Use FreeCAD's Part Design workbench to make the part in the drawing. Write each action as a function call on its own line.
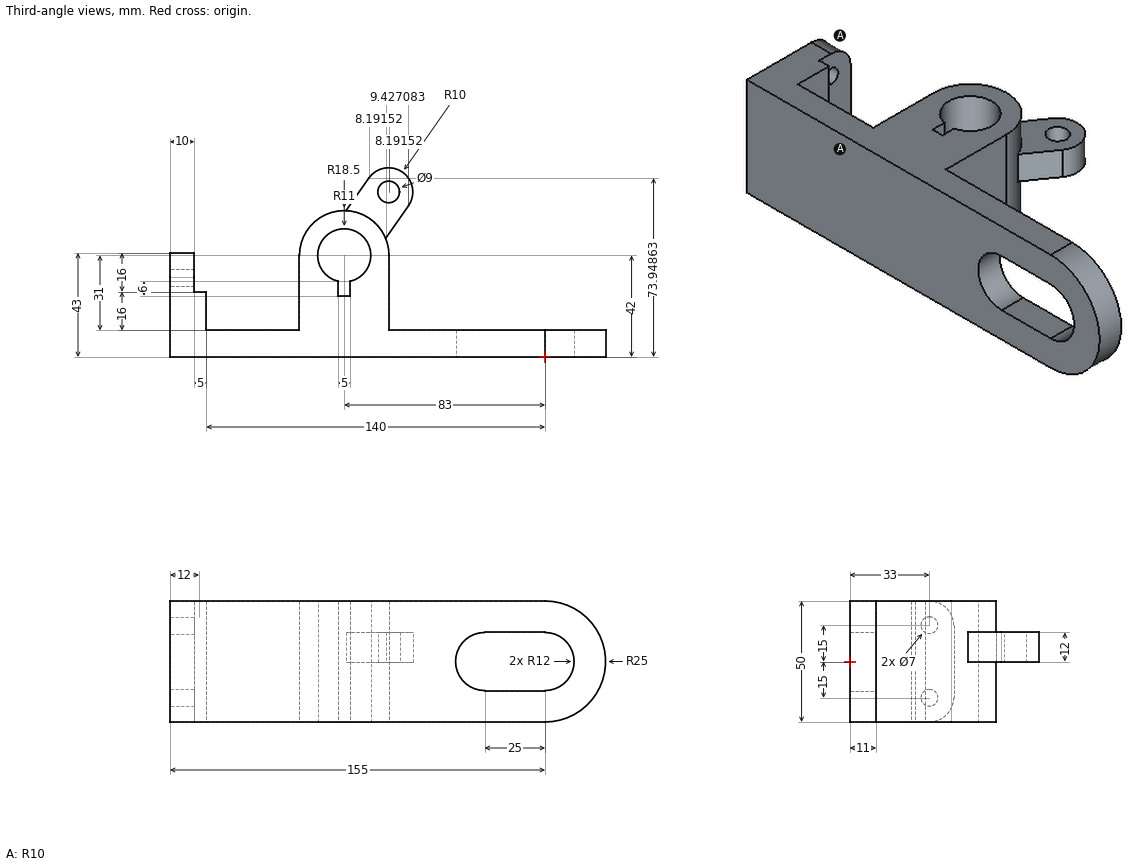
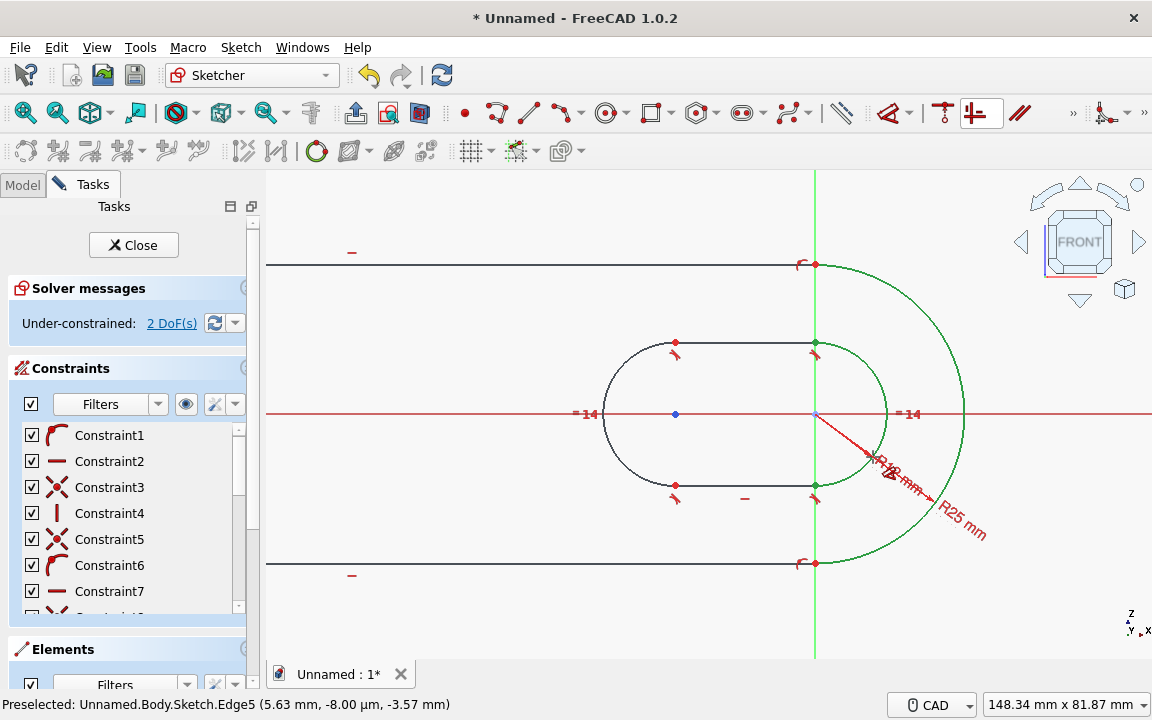
click(773, 486)
click(745, 520)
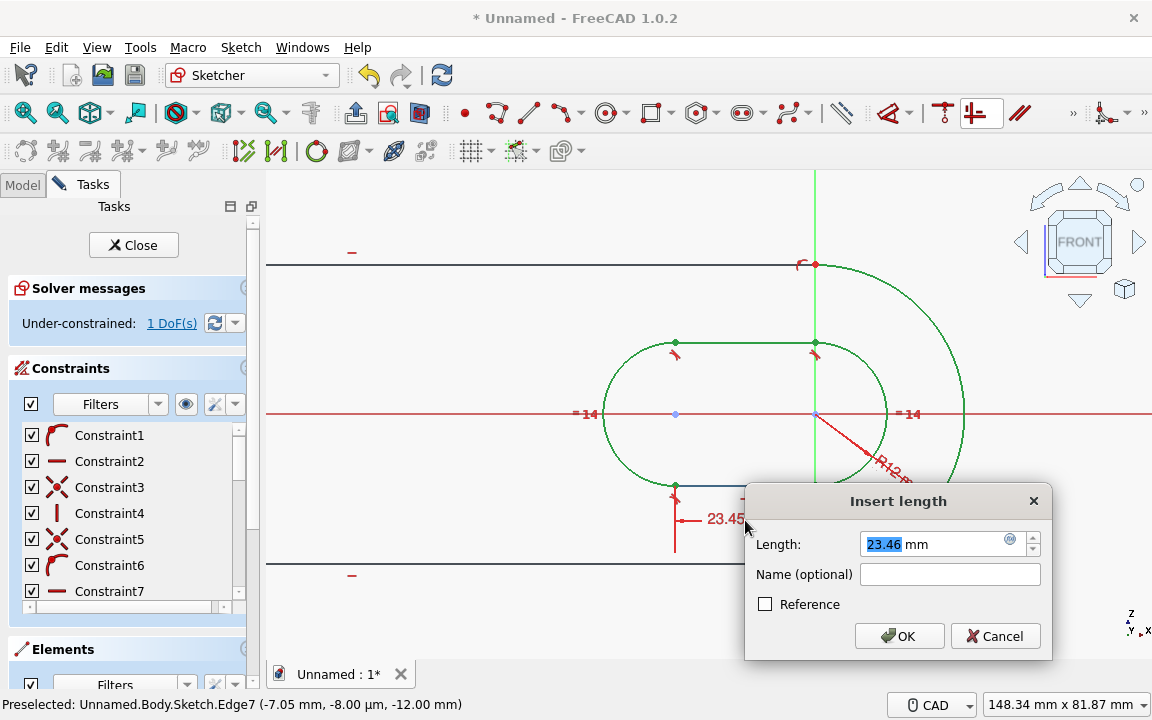
text(25)
key(Return)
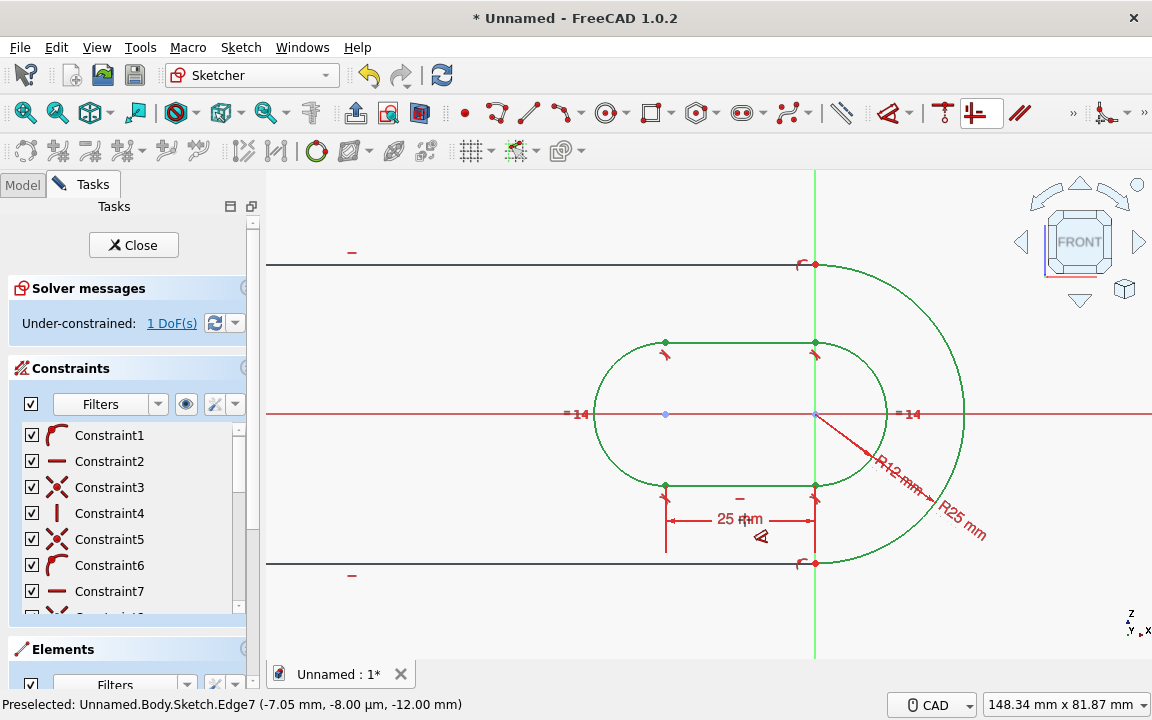
click(537, 564)
click(555, 598)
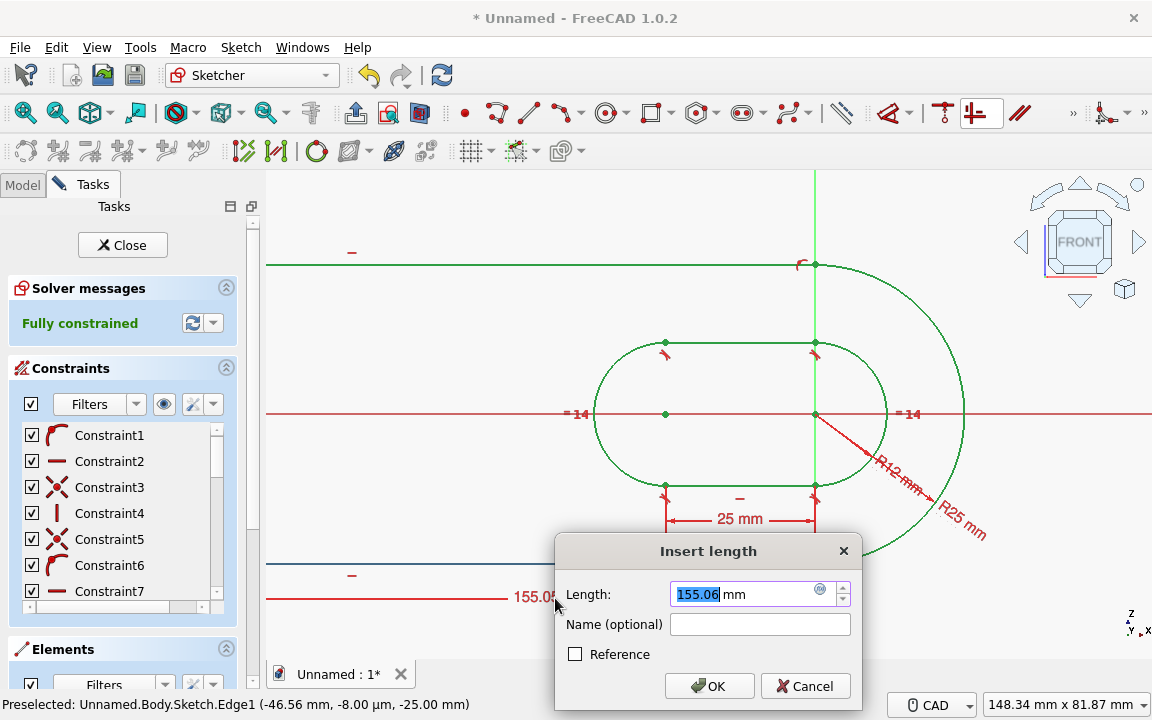
text(155)
key(Return)
key(Escape)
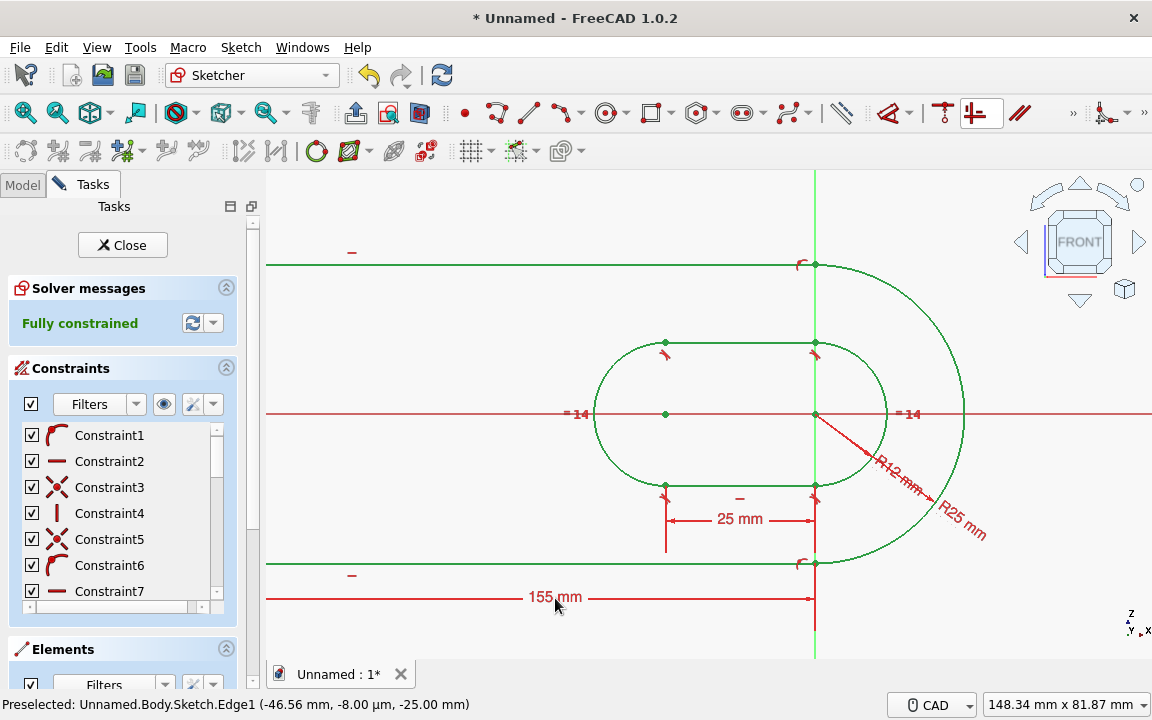
click(123, 245)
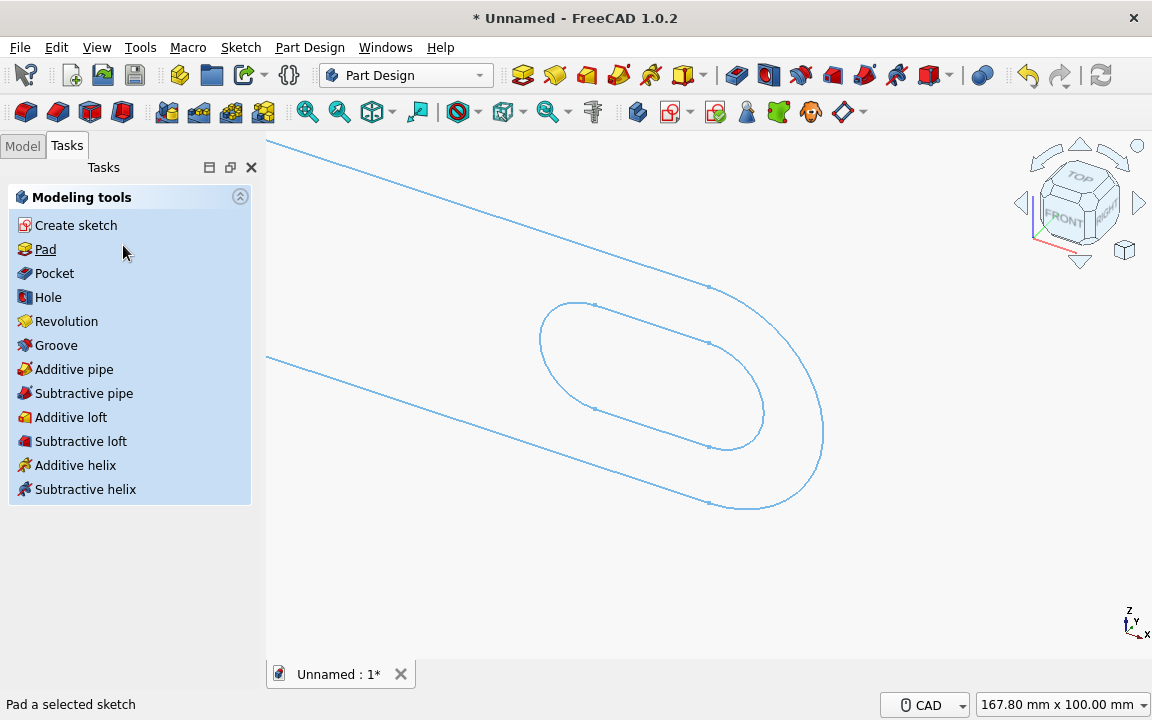
click(524, 76)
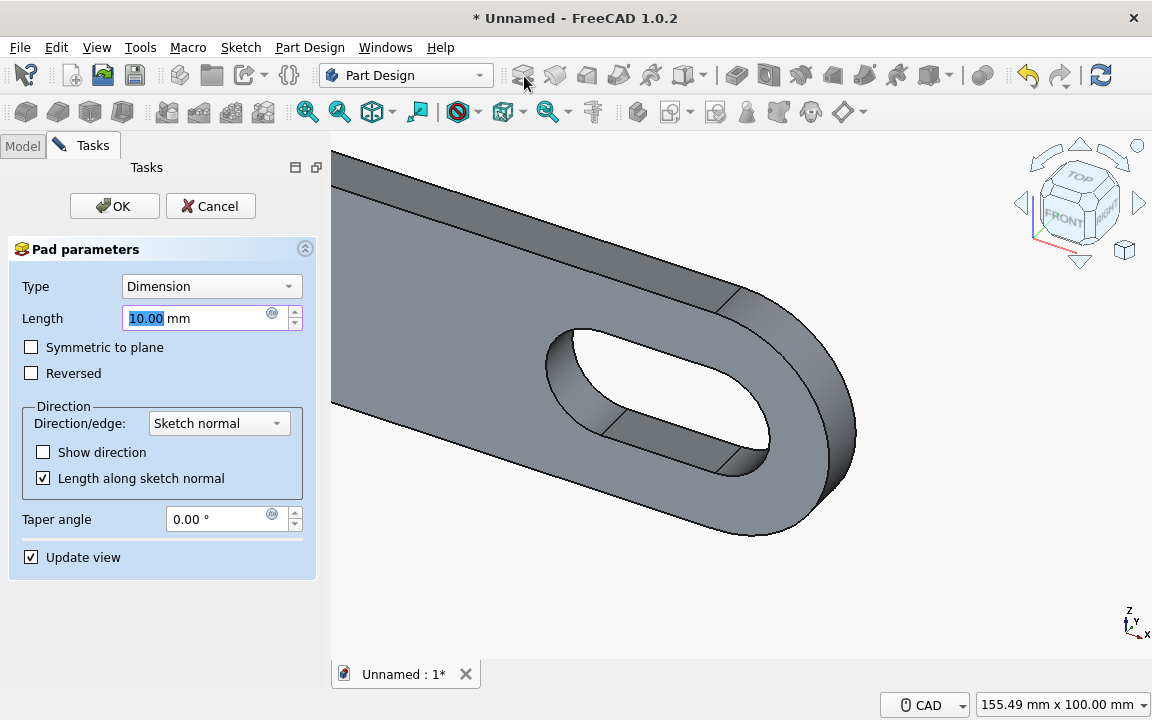
text(11)
key(Tab)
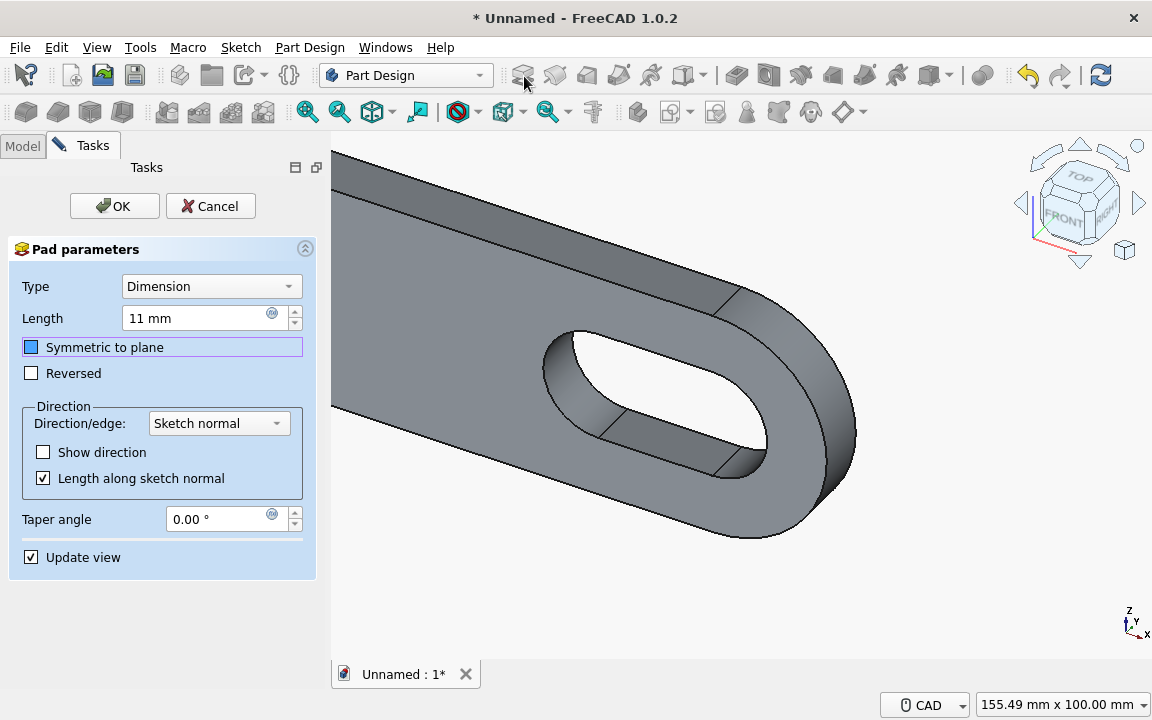
click(30, 373)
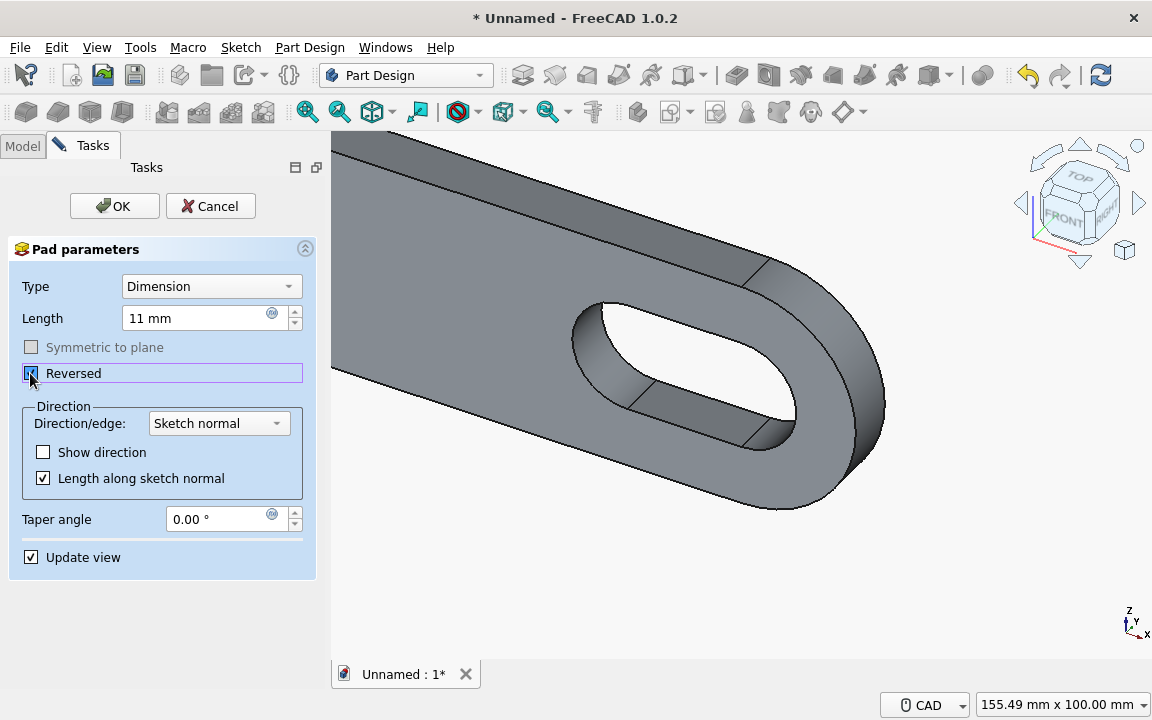
click(115, 206)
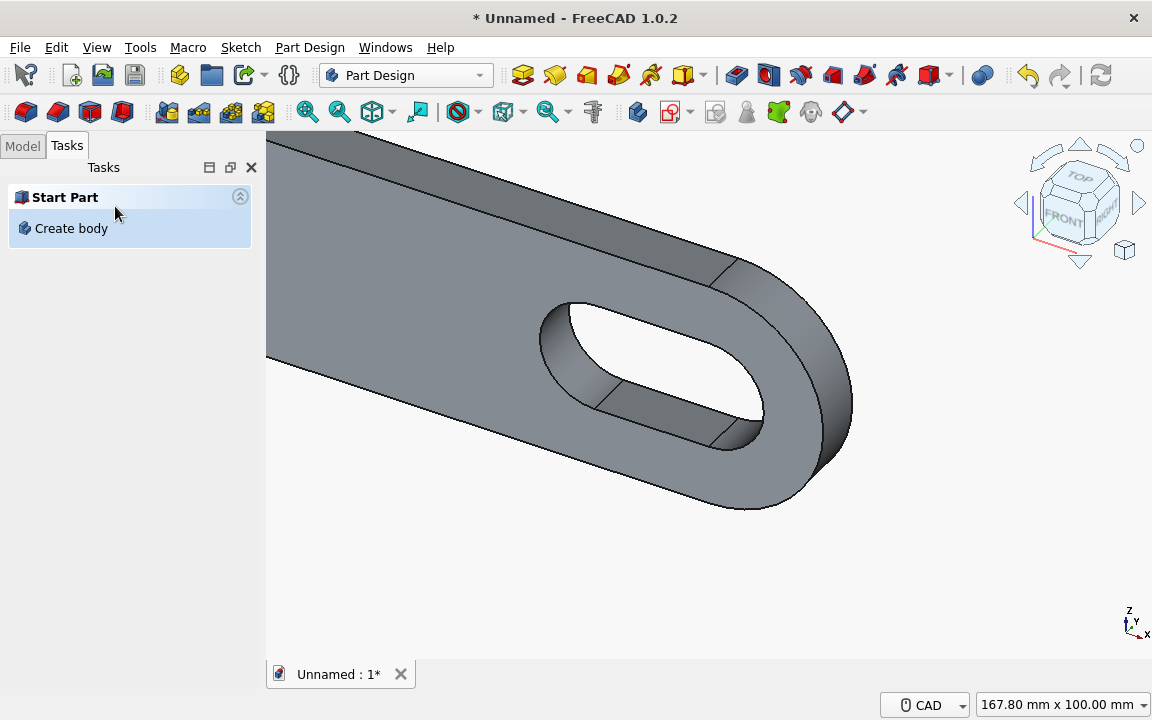
click(308, 112)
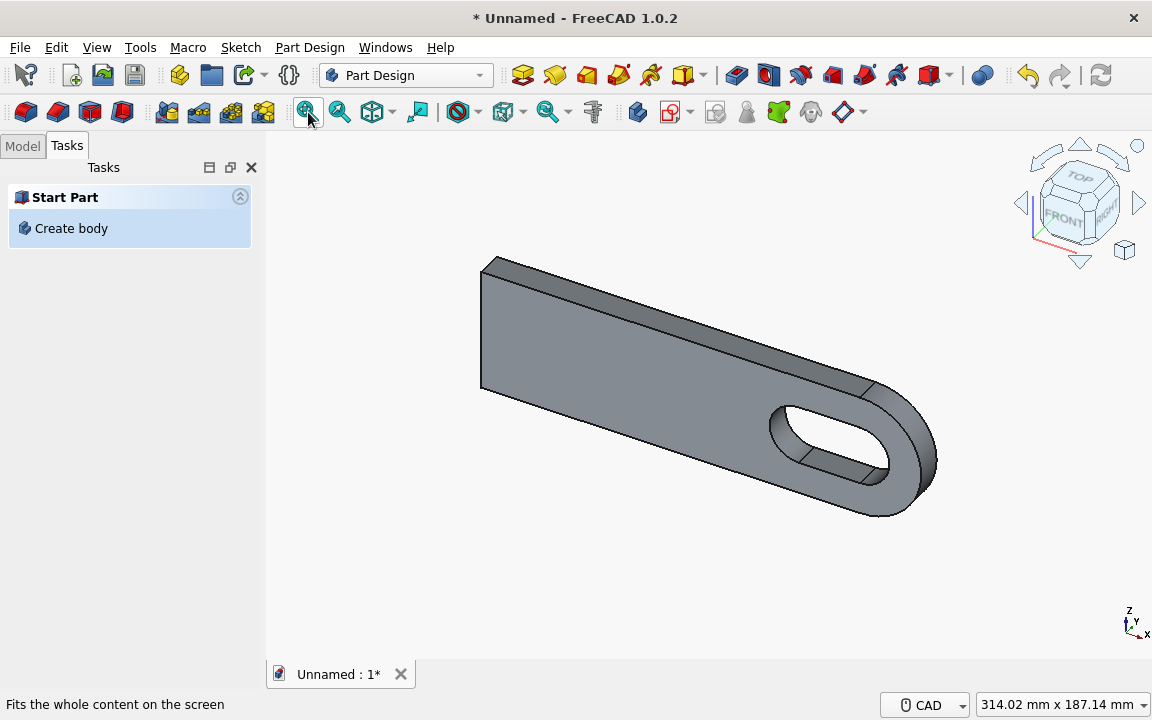
click(841, 380)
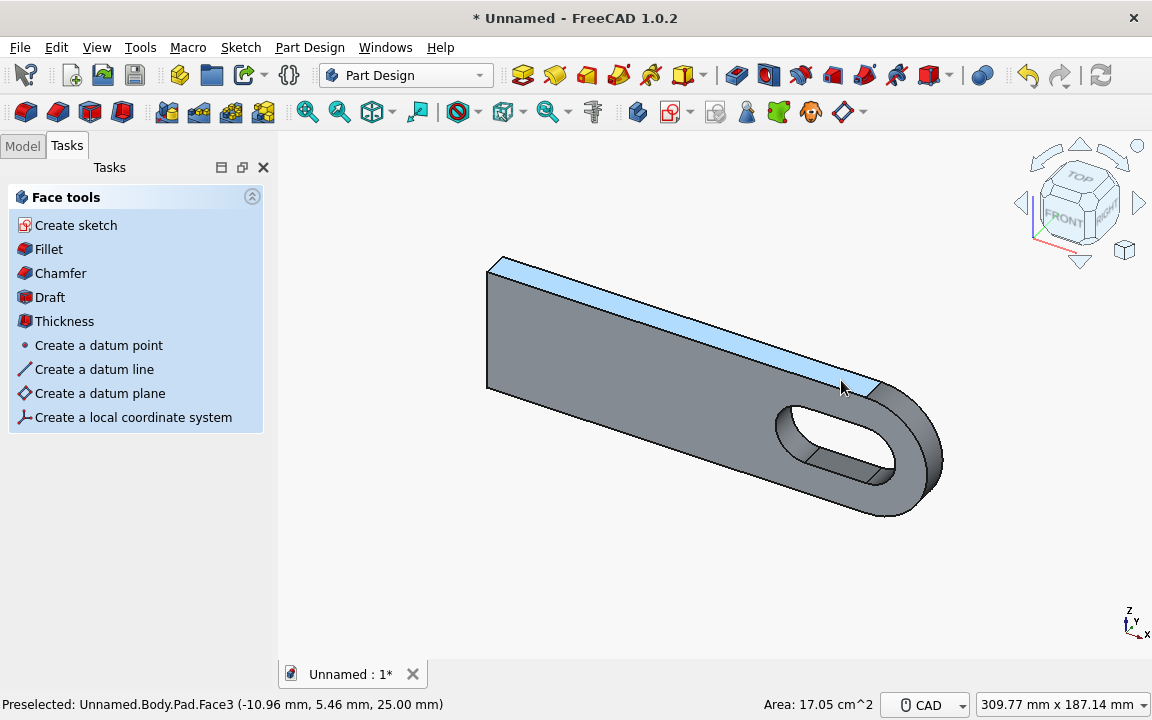
click(670, 112)